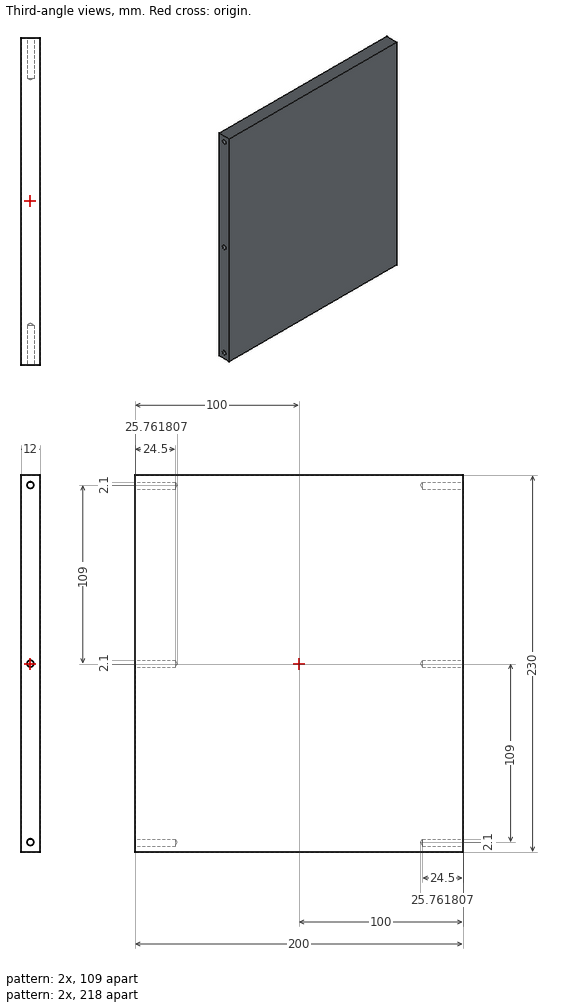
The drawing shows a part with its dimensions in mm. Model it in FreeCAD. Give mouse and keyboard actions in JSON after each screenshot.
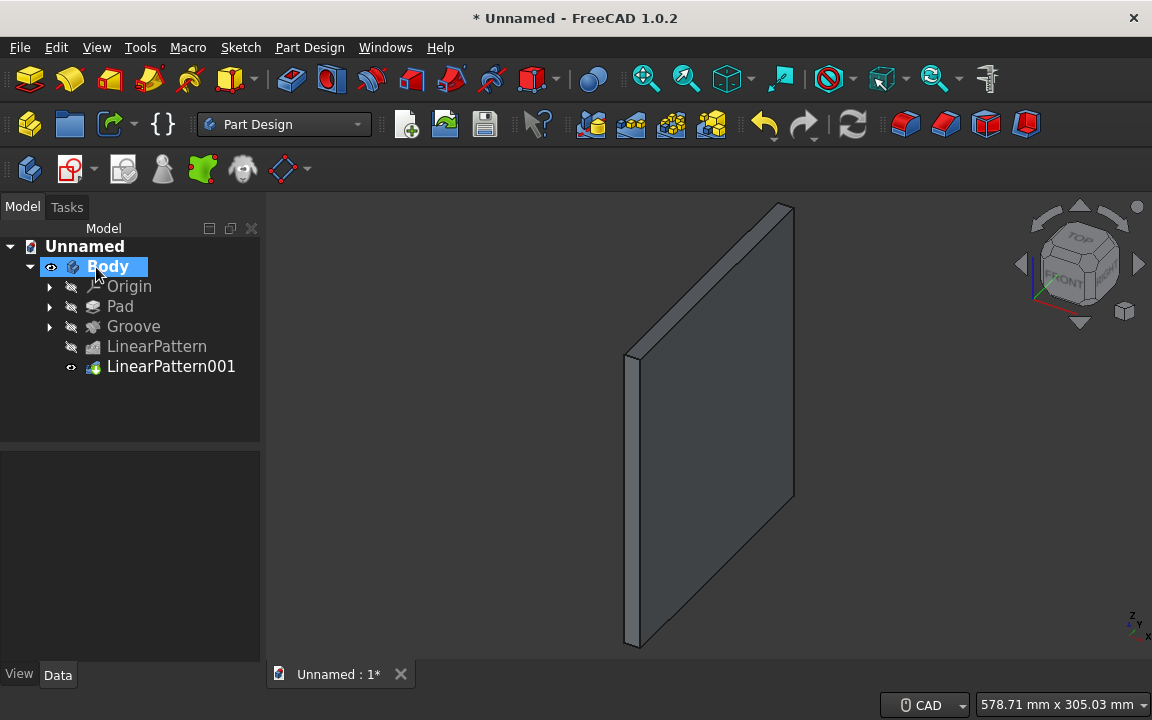
{"action": "left_click", "coordinate": [116, 327]}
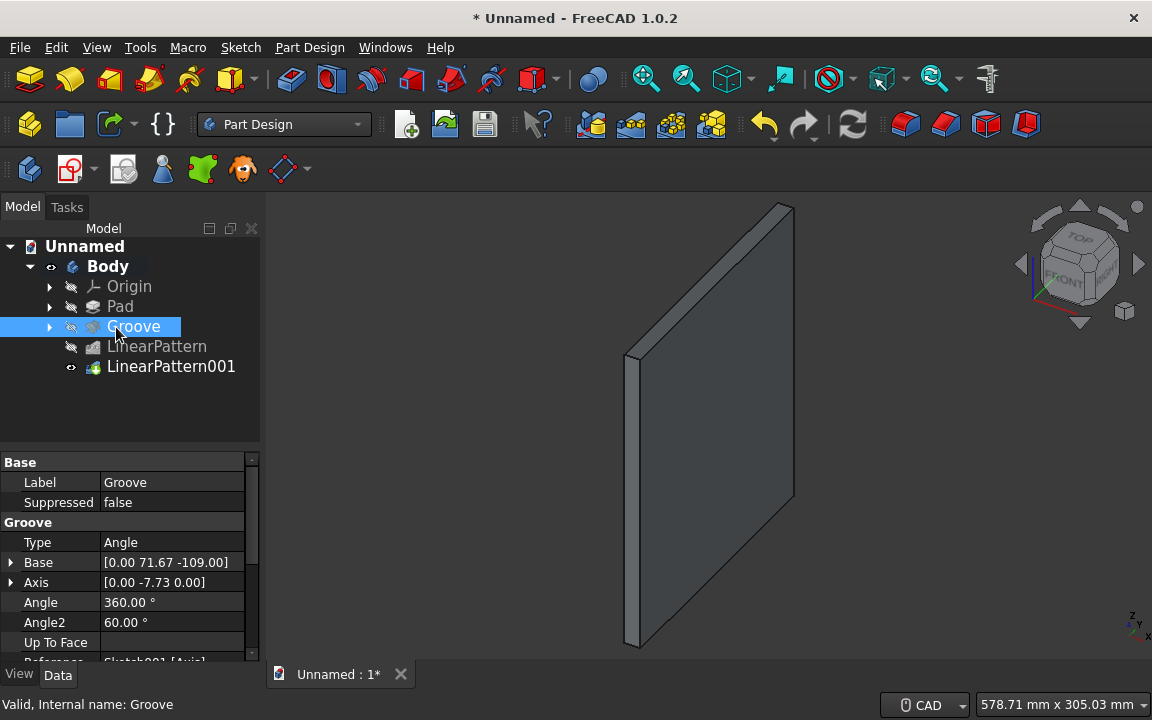
{"action": "left_click", "coordinate": [592, 124]}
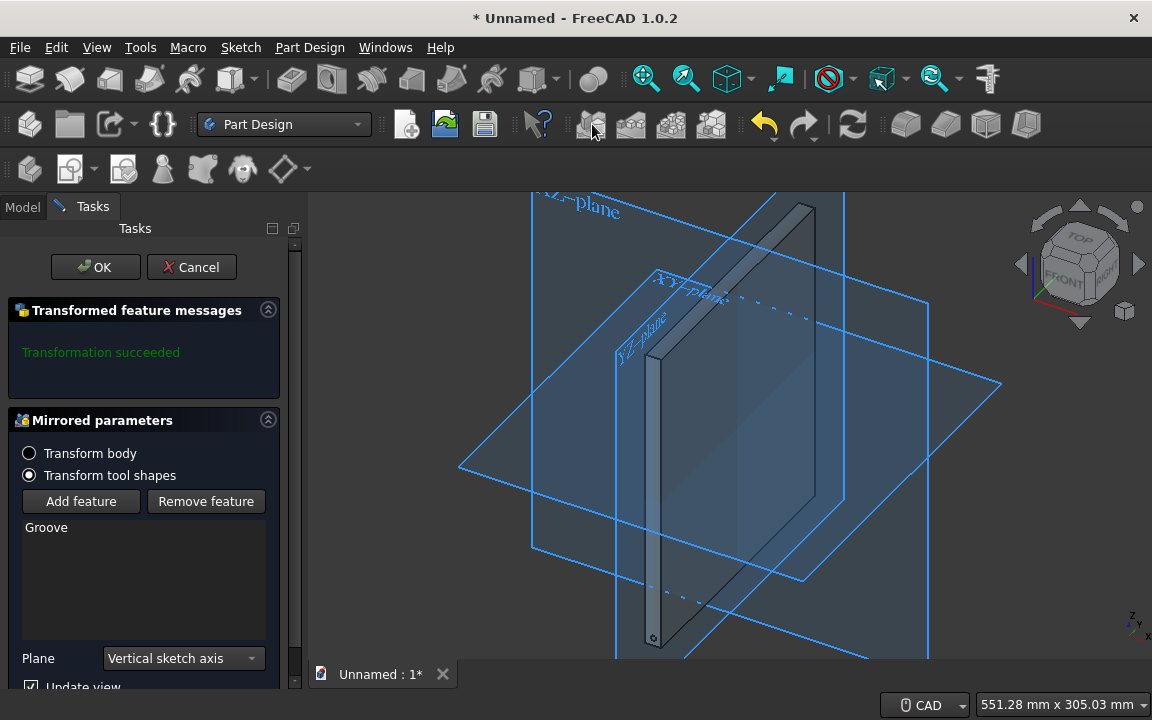
{"action": "left_click", "coordinate": [184, 658]}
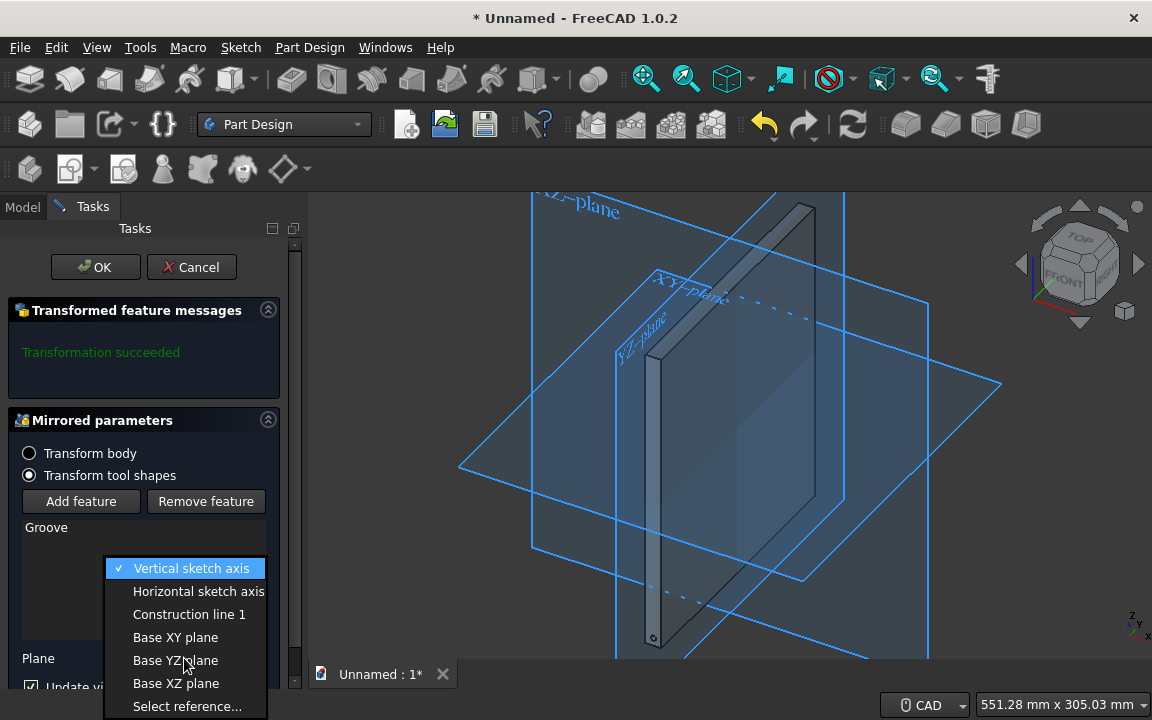
{"action": "left_click", "coordinate": [184, 684]}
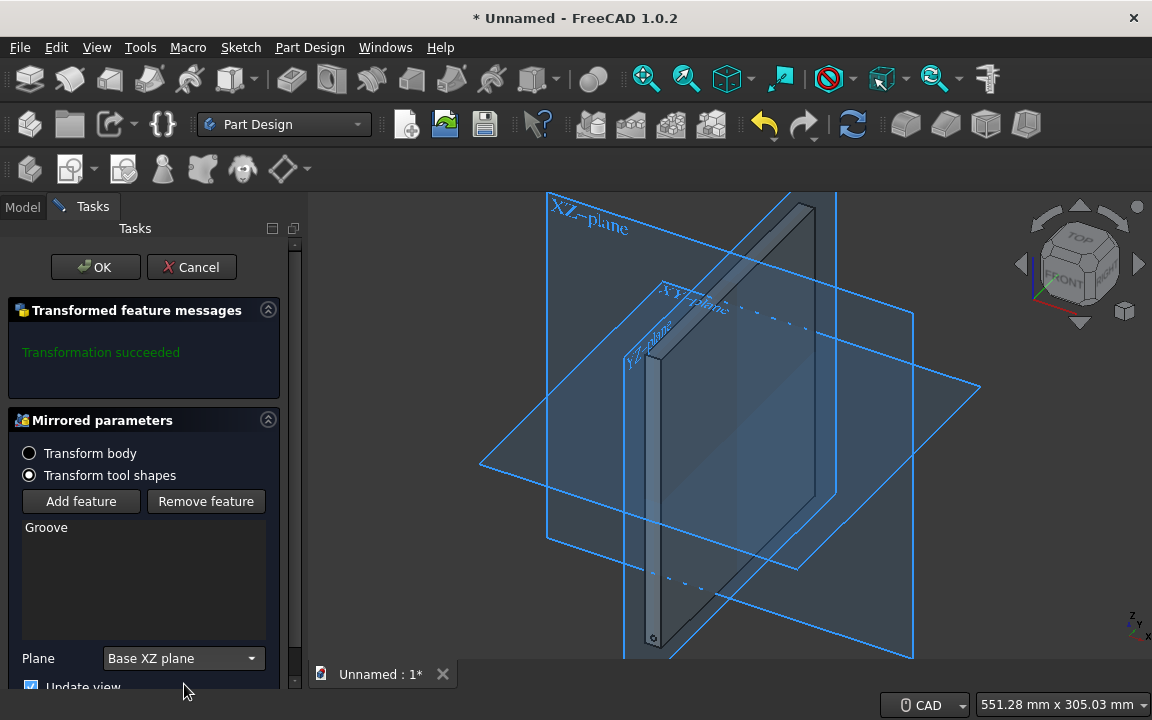
{"action": "left_click", "coordinate": [96, 267]}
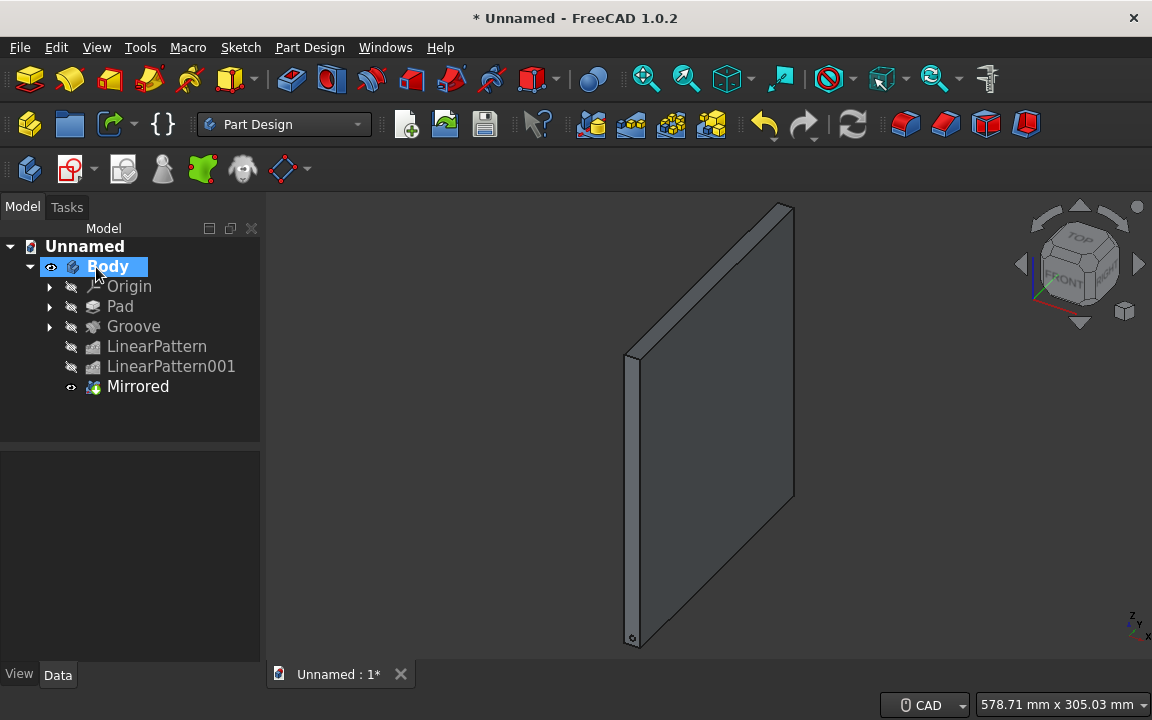
{"action": "left_click", "coordinate": [70, 170]}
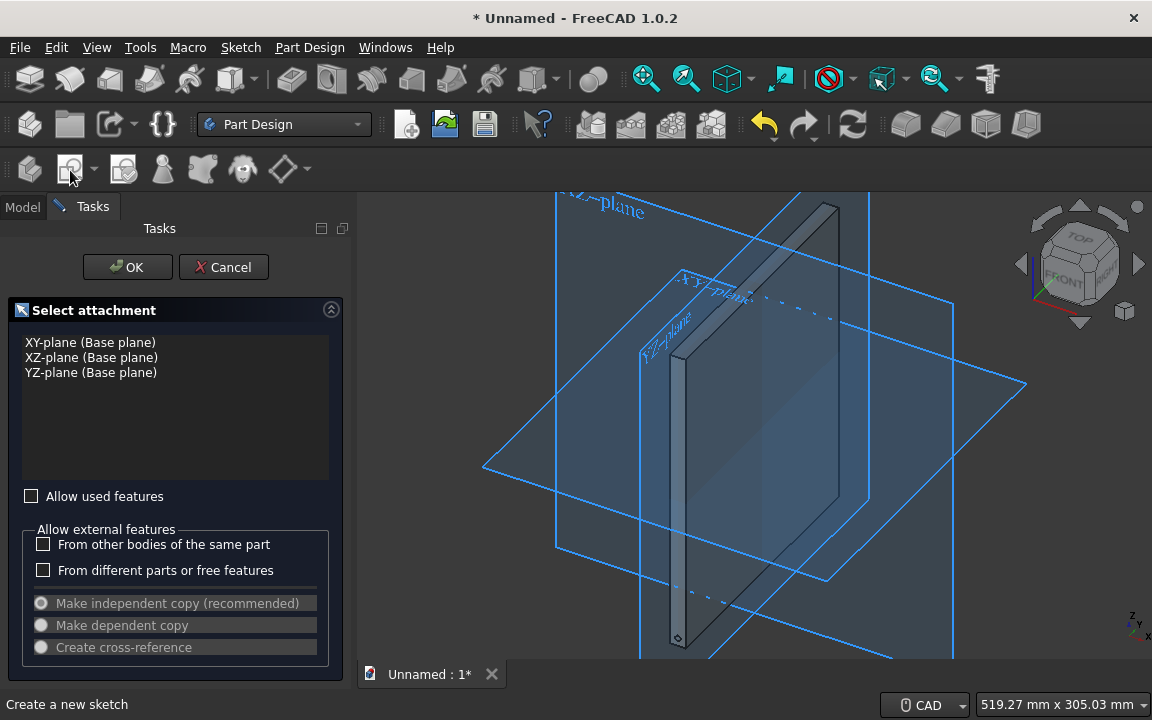
{"action": "left_click", "coordinate": [82, 372]}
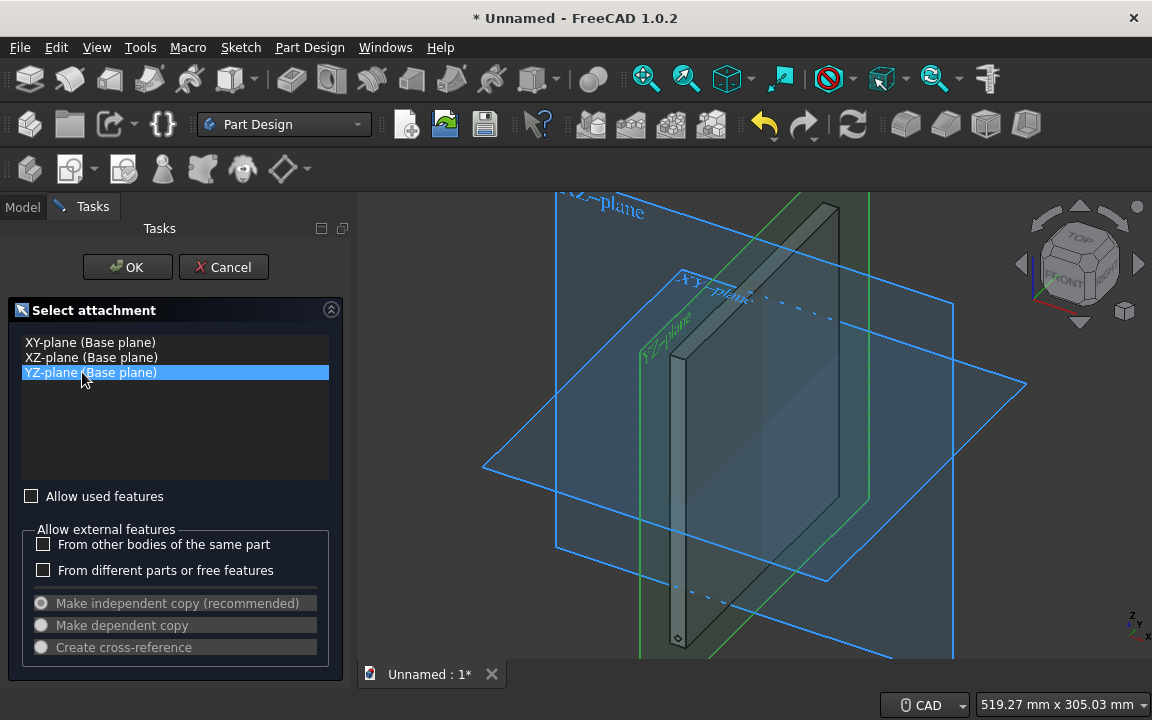
{"action": "left_click", "coordinate": [128, 267]}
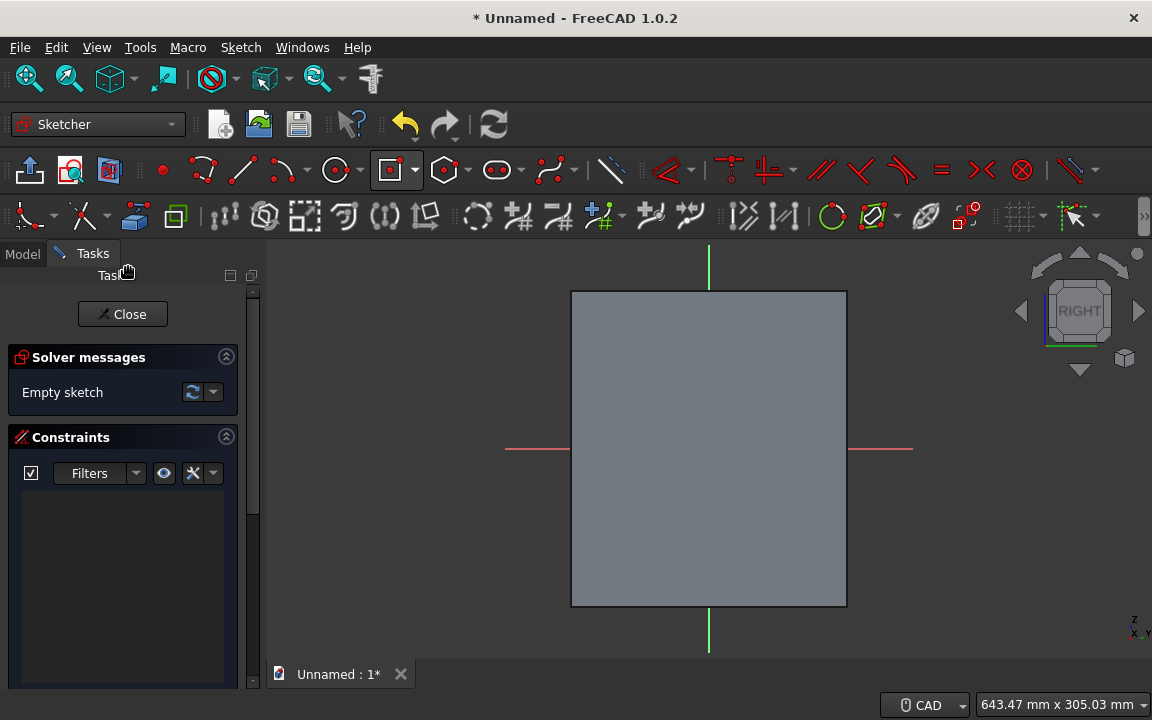
{"action": "left_click", "coordinate": [110, 170]}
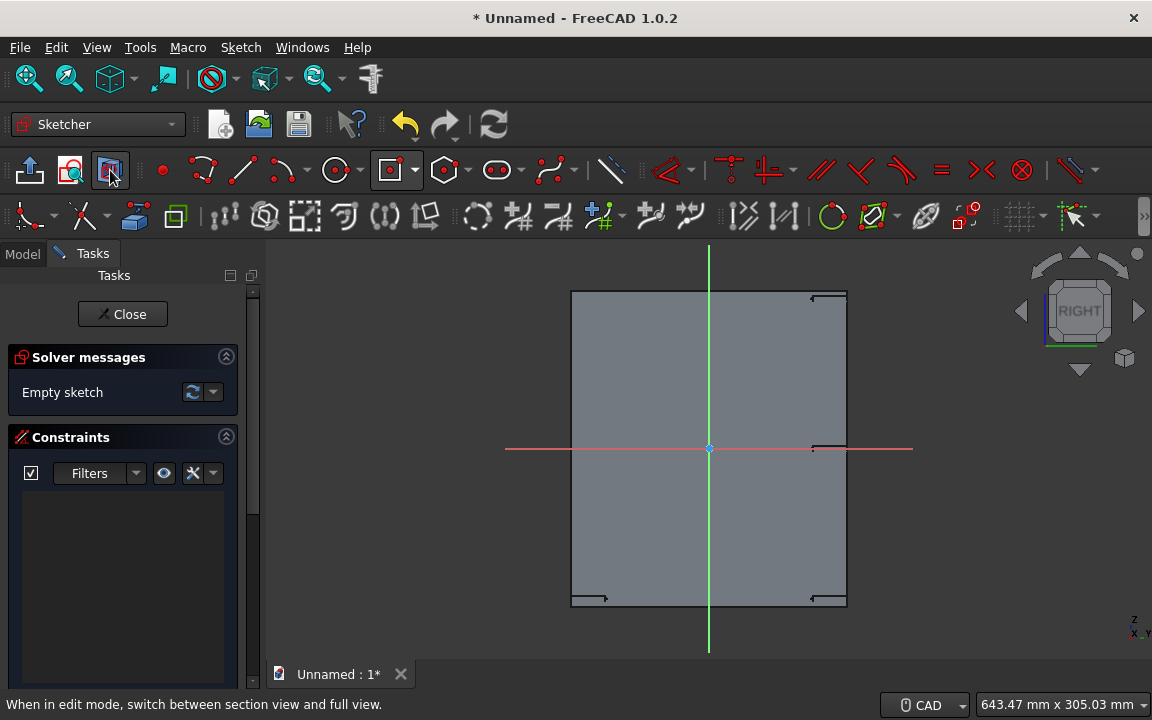
{"action": "scroll", "coordinate": [585, 447], "scroll_direction": "up", "scroll_amount": 13}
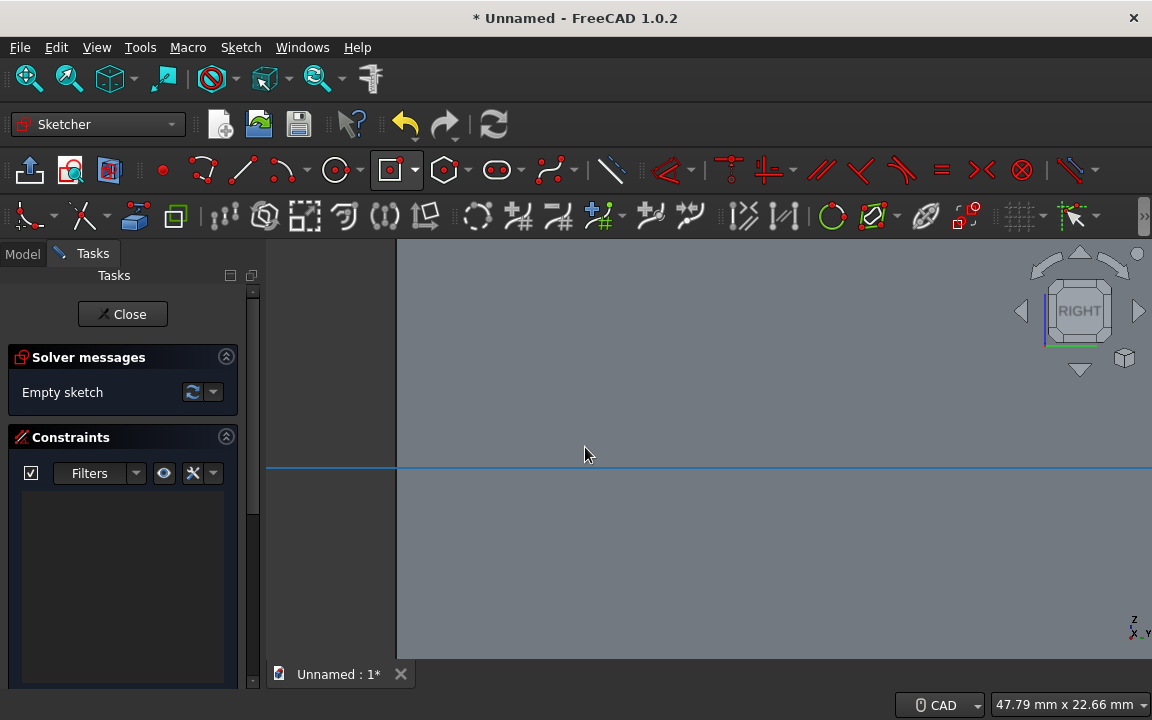
{"action": "left_click", "coordinate": [204, 170]}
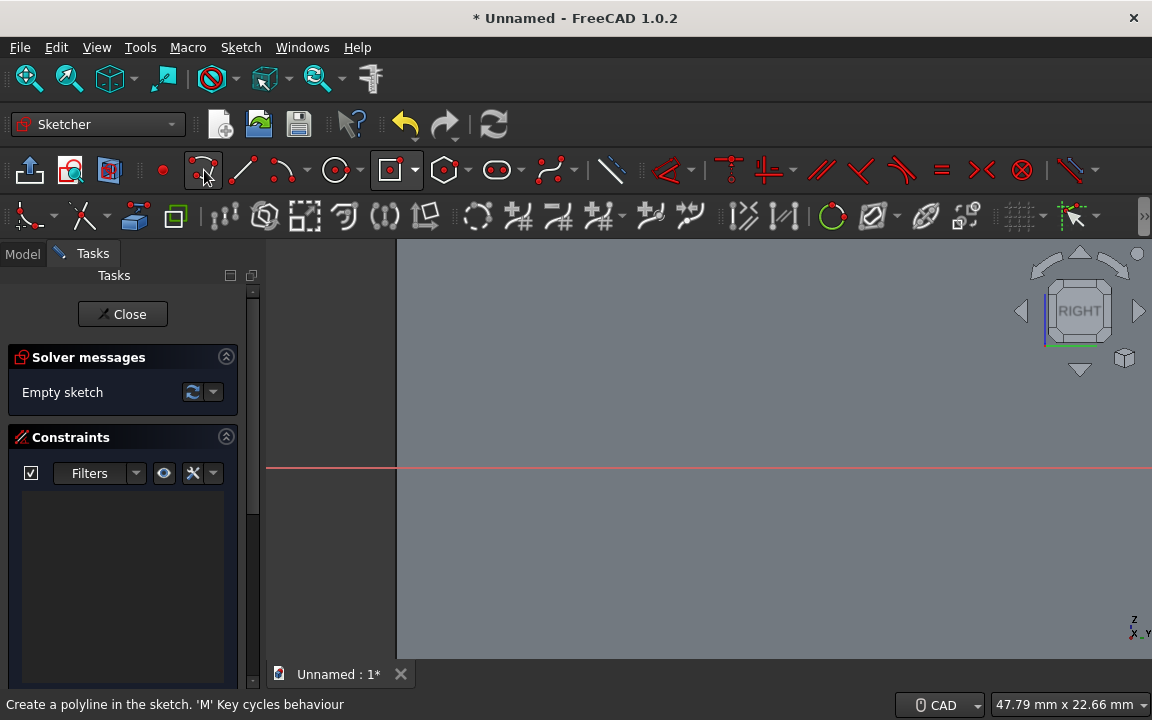
{"action": "left_click", "coordinate": [874, 468]}
{"action": "left_click", "coordinate": [850, 429]}
{"action": "left_click", "coordinate": [396, 429]}
{"action": "left_click", "coordinate": [396, 459]}
{"action": "left_click", "coordinate": [874, 468]}
{"action": "key", "text": "Escape"}
{"action": "key", "text": "Escape"}